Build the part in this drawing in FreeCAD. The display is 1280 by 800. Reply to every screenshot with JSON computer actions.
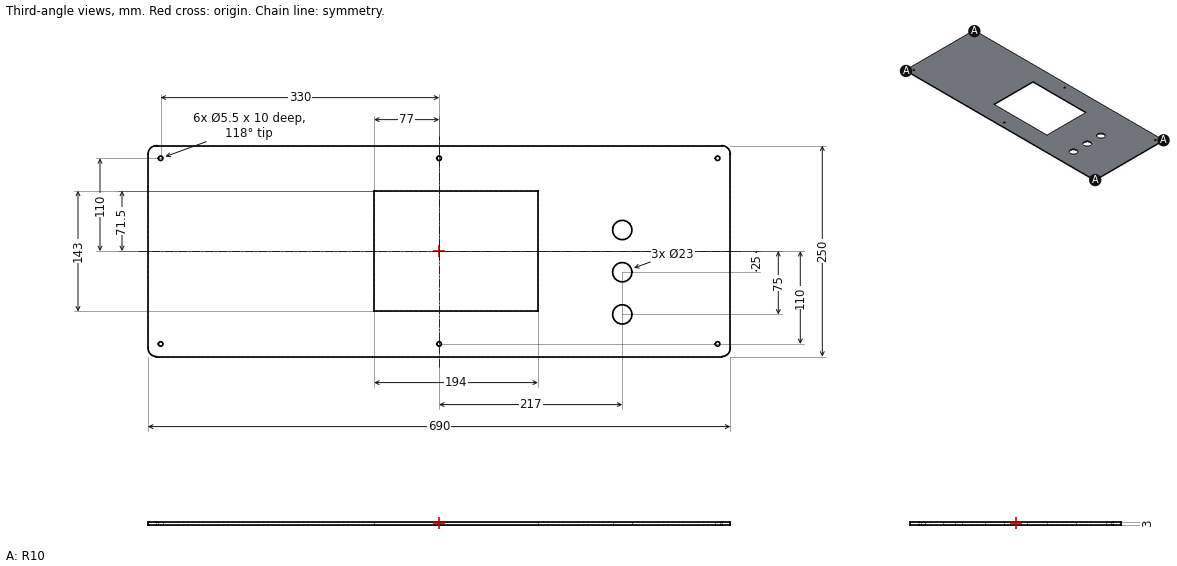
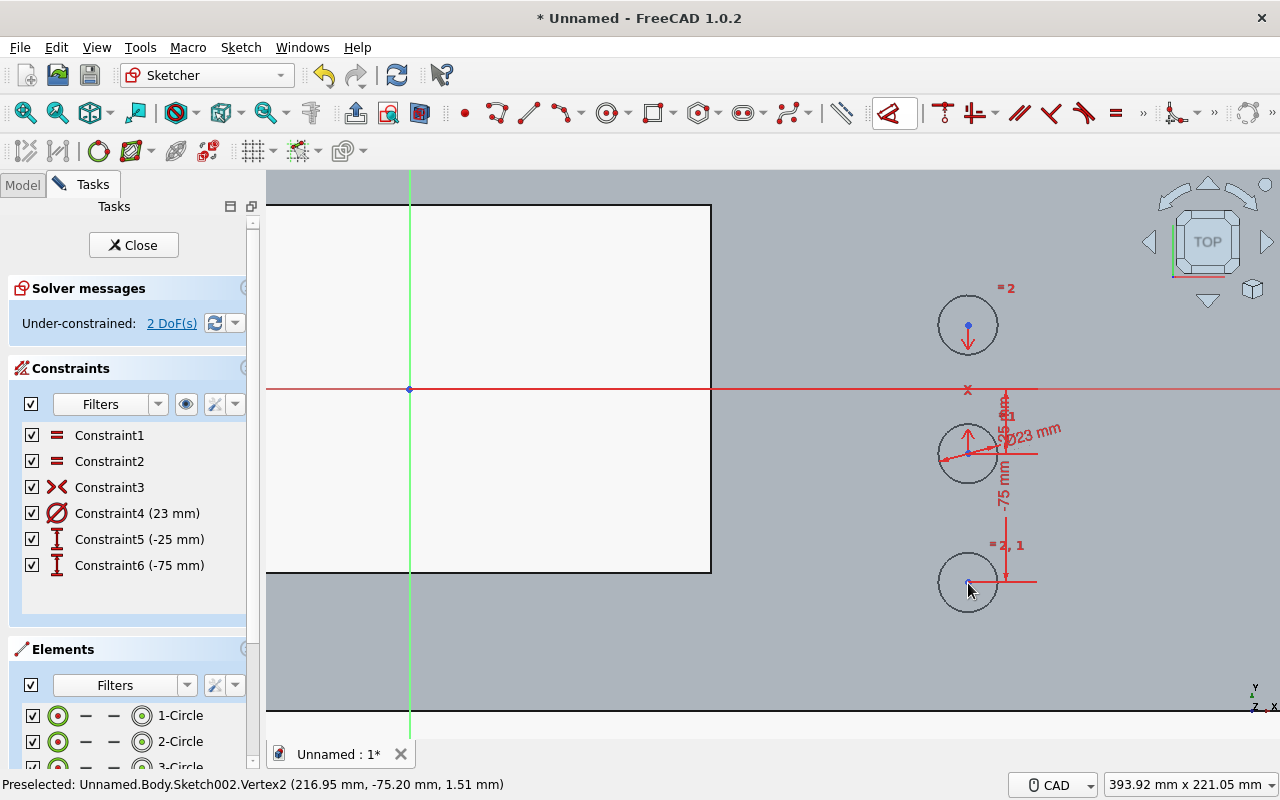
{"action": "left_click", "coordinate": [968, 454]}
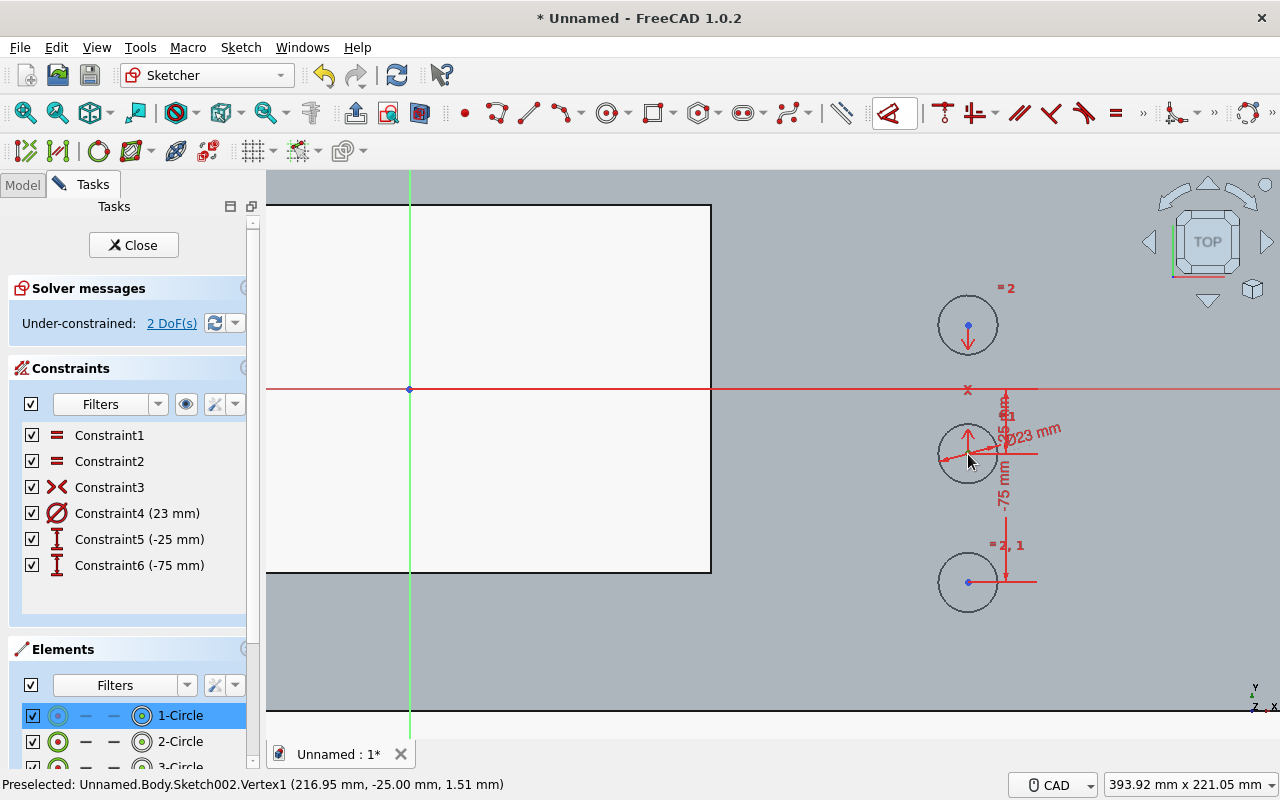
{"action": "left_click", "coordinate": [912, 114]}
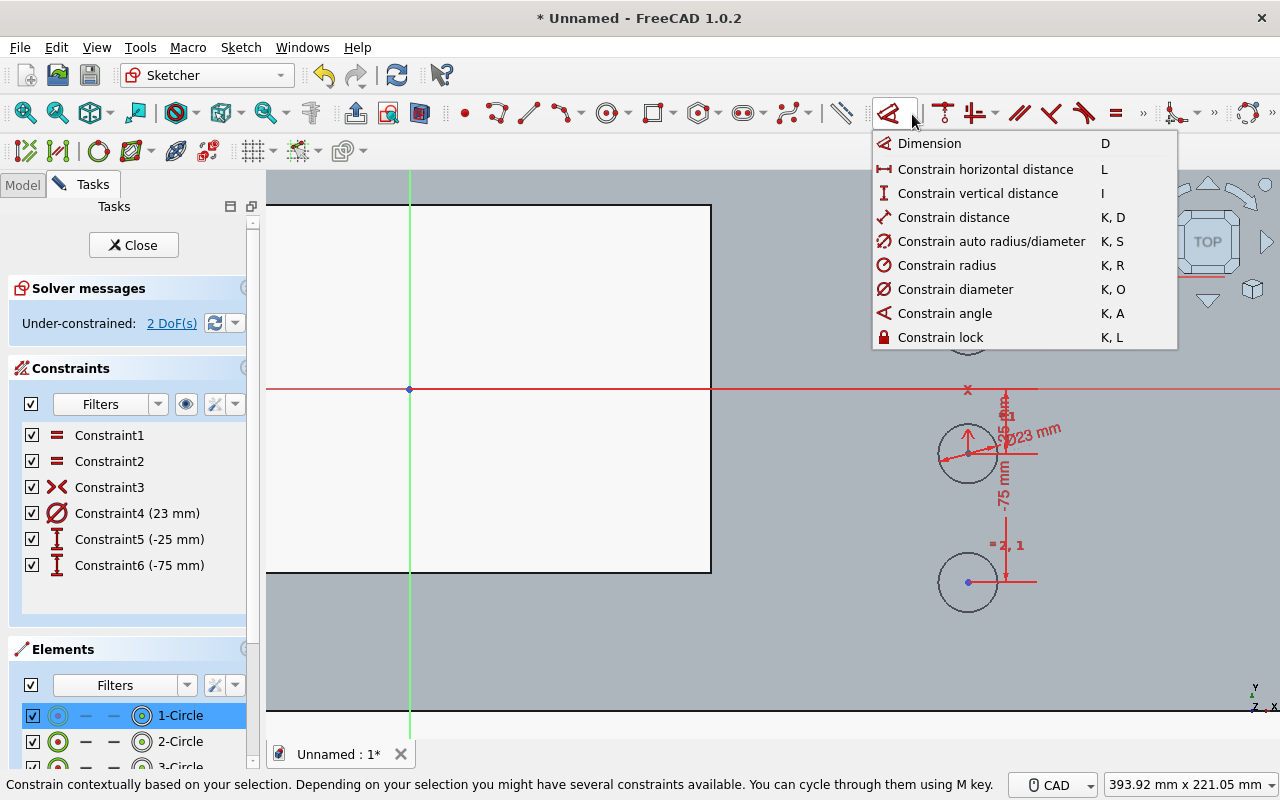
{"action": "left_click", "coordinate": [1025, 169]}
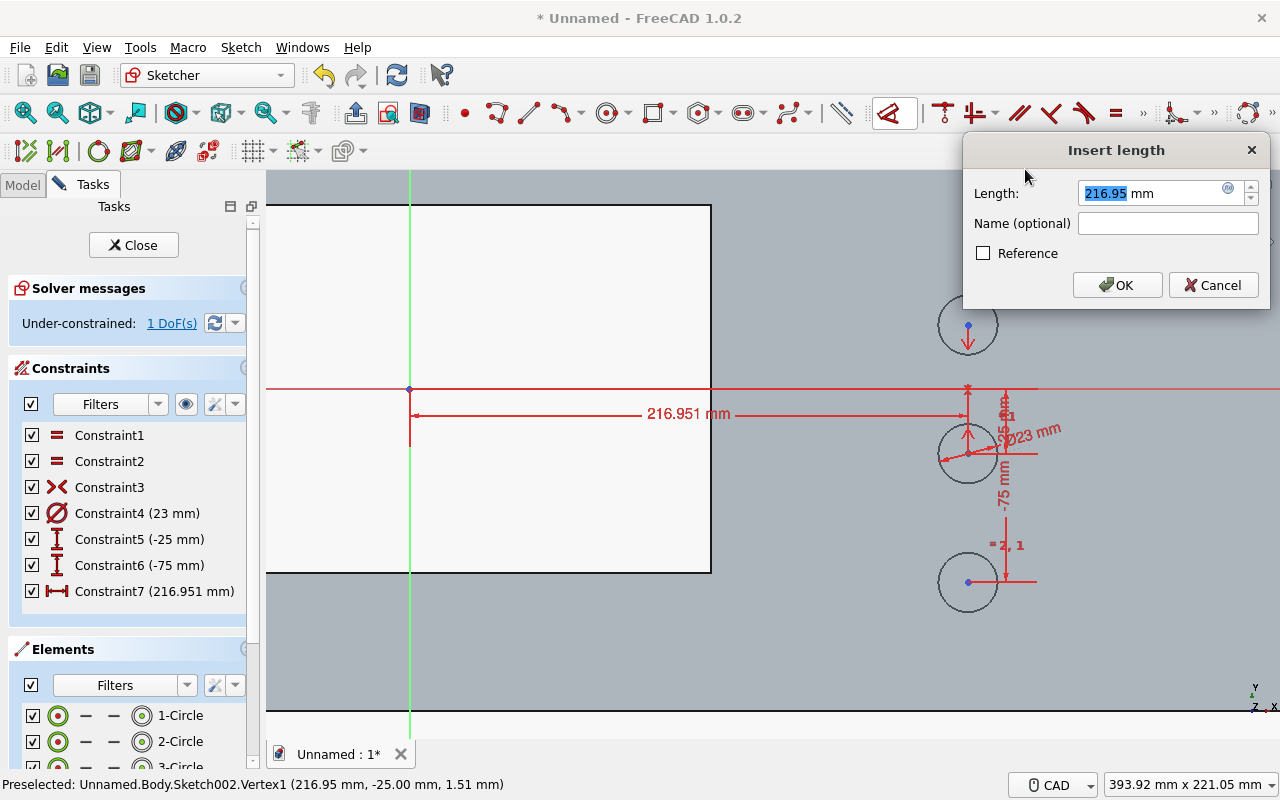
{"action": "type", "text": "217"}
{"action": "key", "text": "Return"}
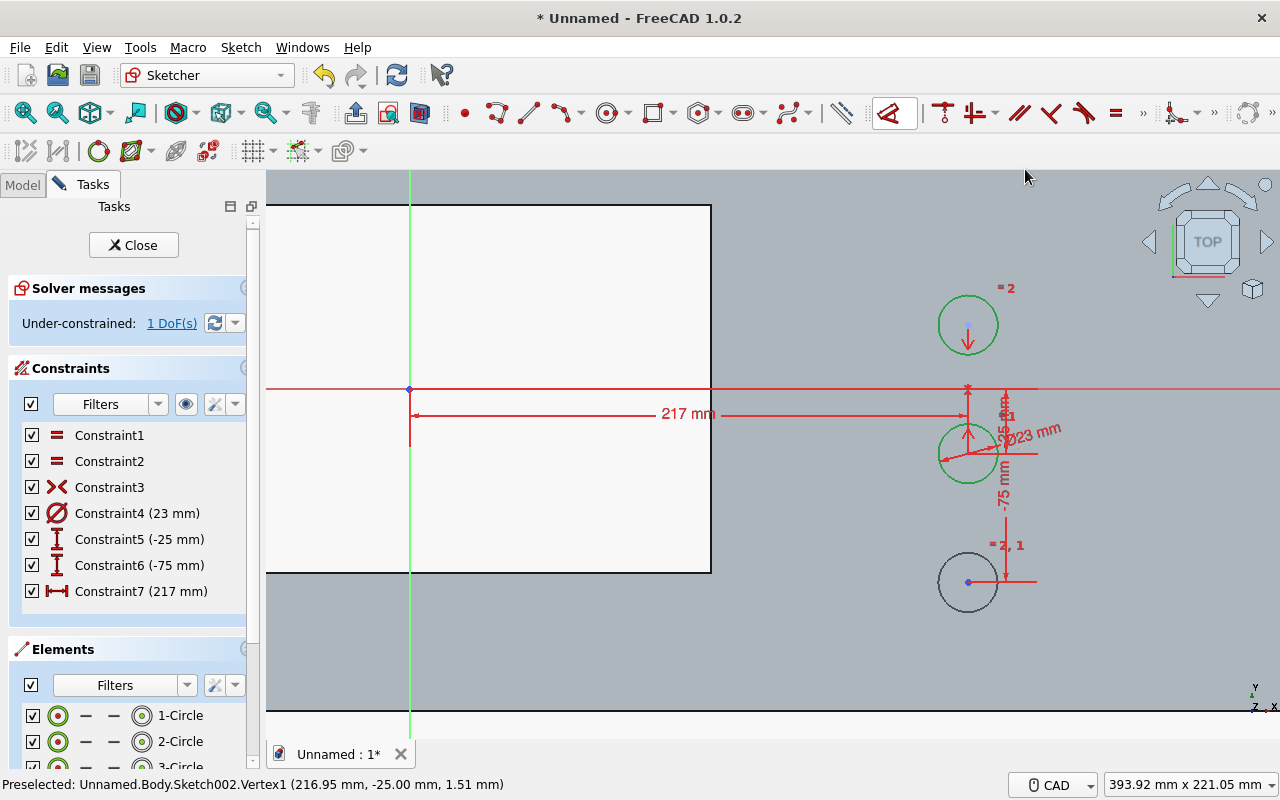
{"action": "left_click", "coordinate": [968, 582]}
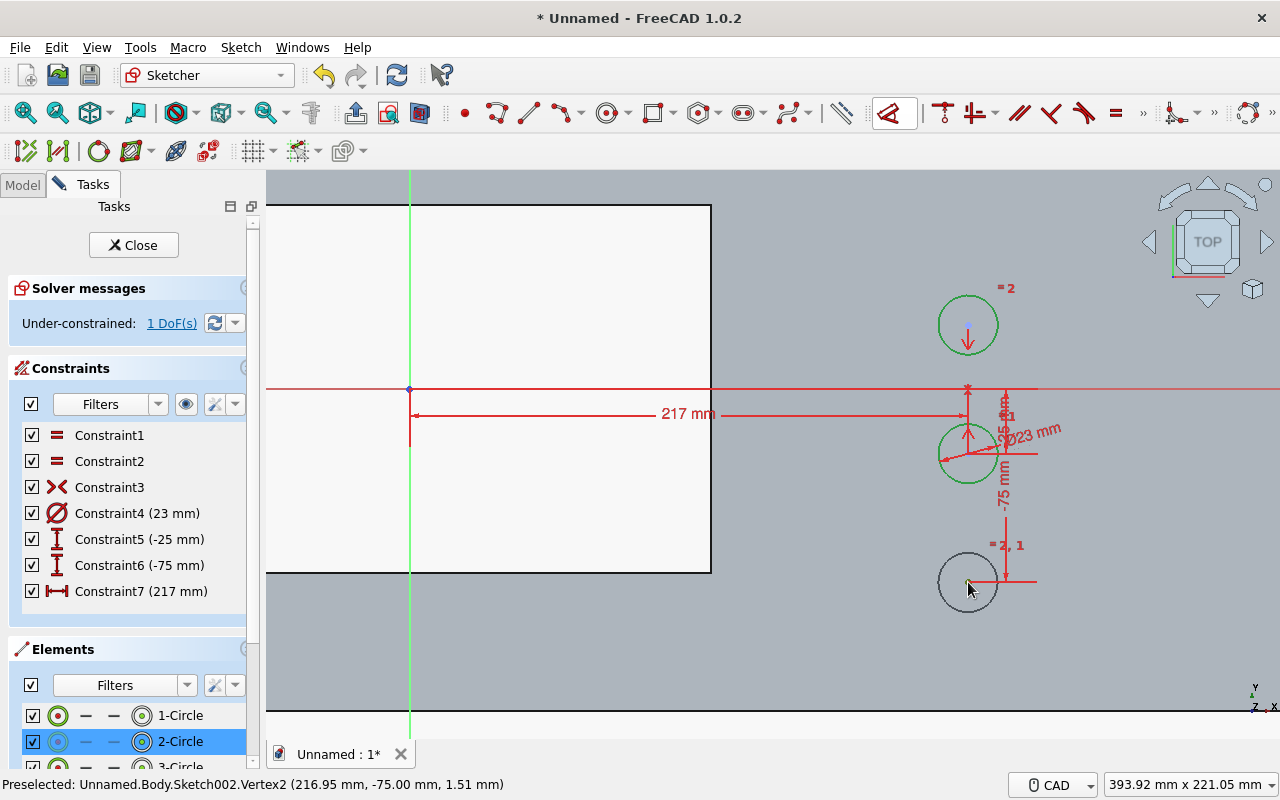
{"action": "key", "text": "l"}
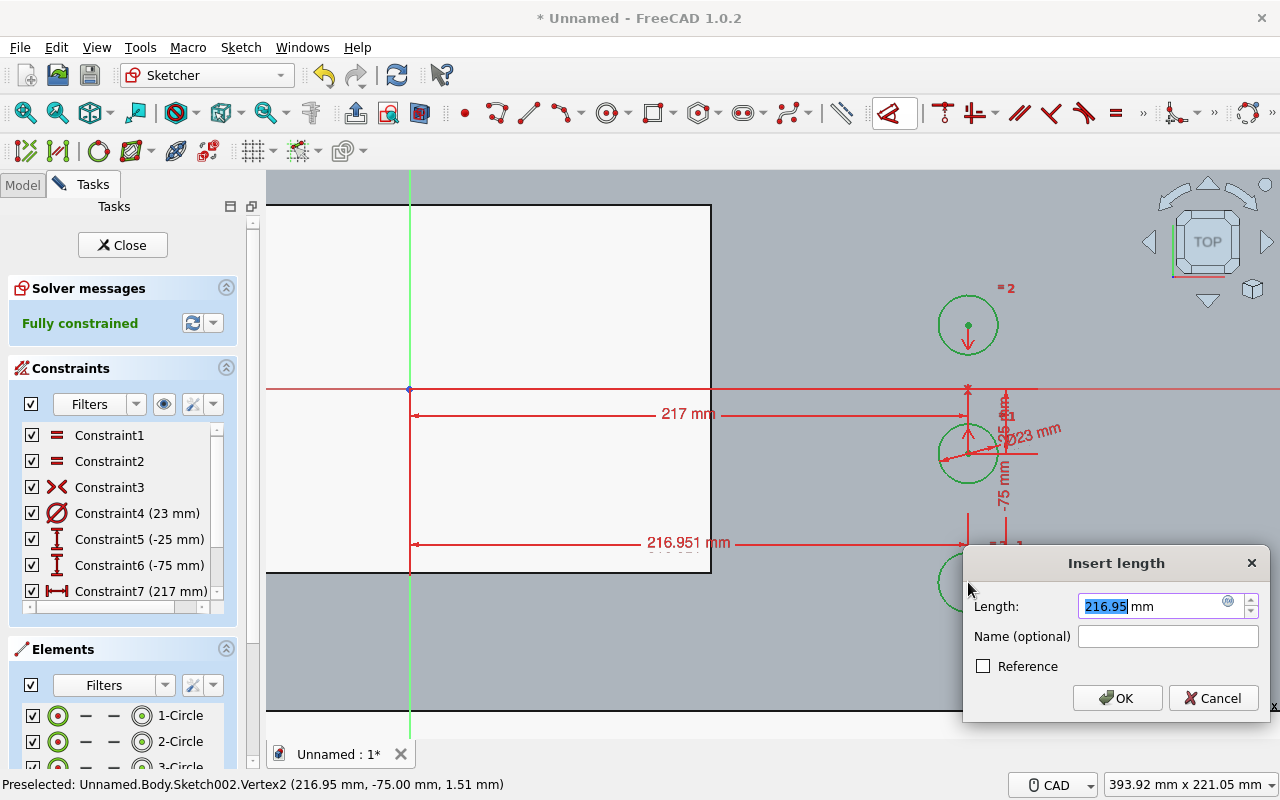
{"action": "type", "text": "217"}
{"action": "key", "text": "Return"}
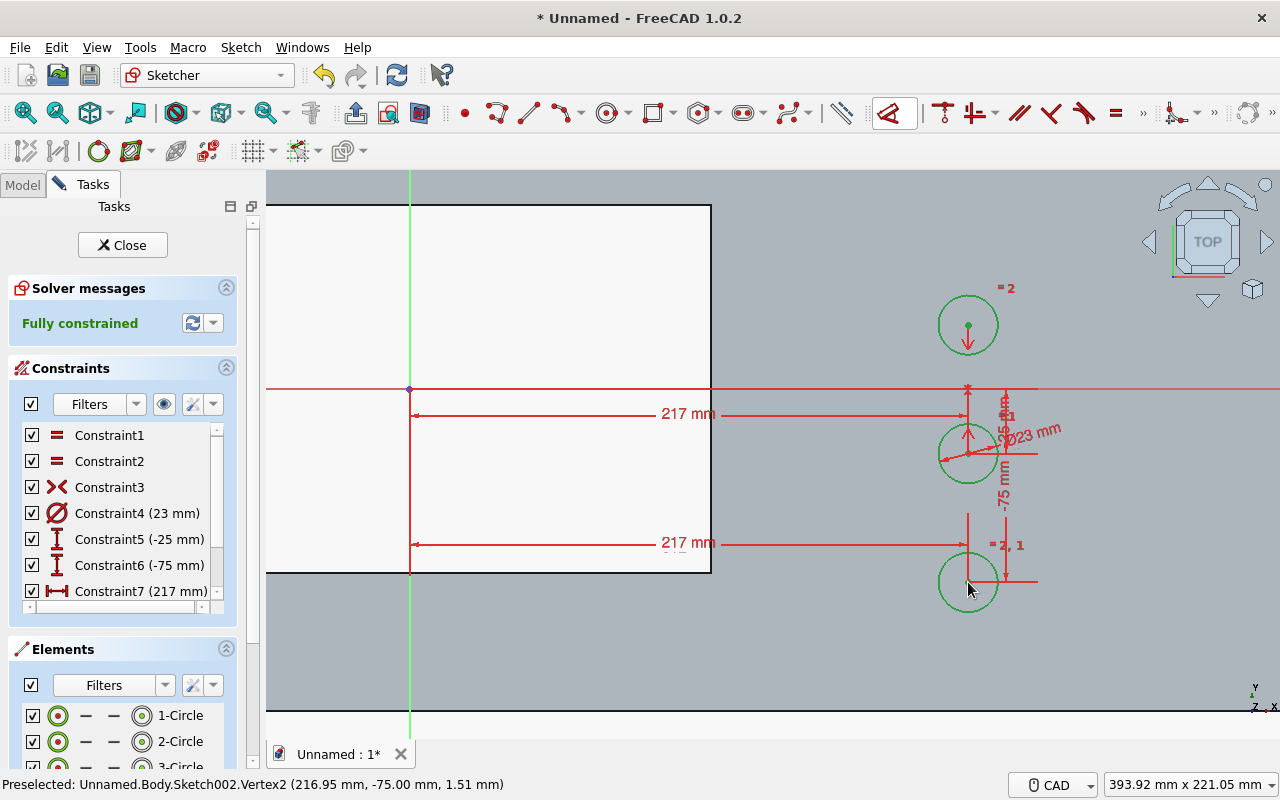
{"action": "left_click", "coordinate": [123, 245]}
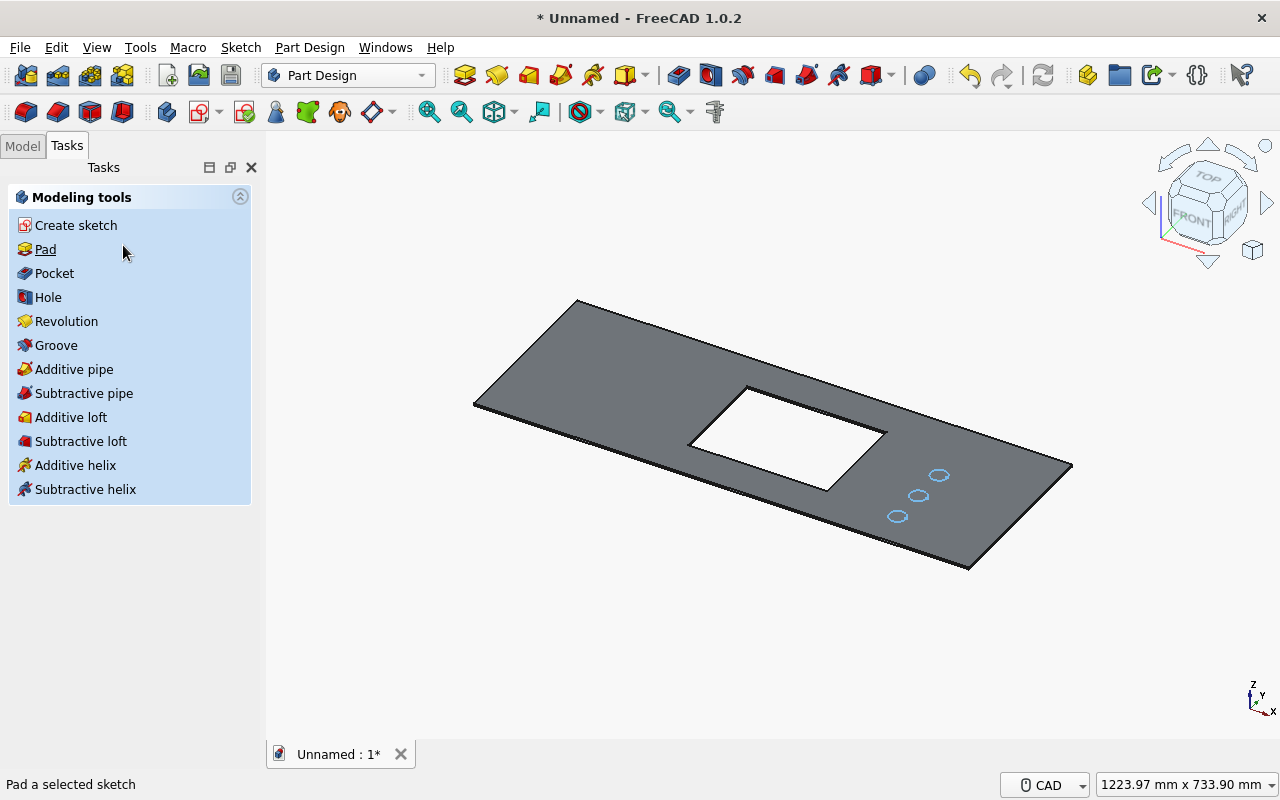
{"action": "left_click", "coordinate": [680, 76]}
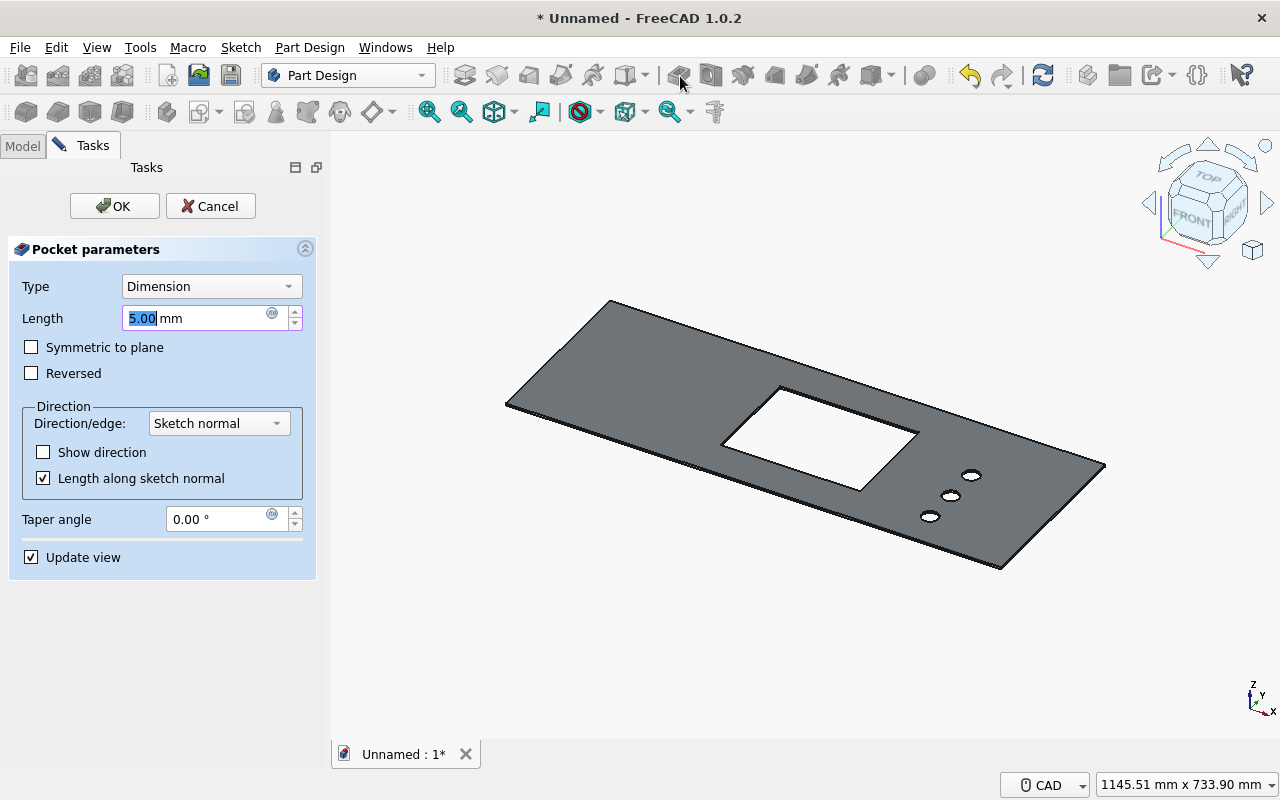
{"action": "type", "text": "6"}
{"action": "key", "text": "Tab"}